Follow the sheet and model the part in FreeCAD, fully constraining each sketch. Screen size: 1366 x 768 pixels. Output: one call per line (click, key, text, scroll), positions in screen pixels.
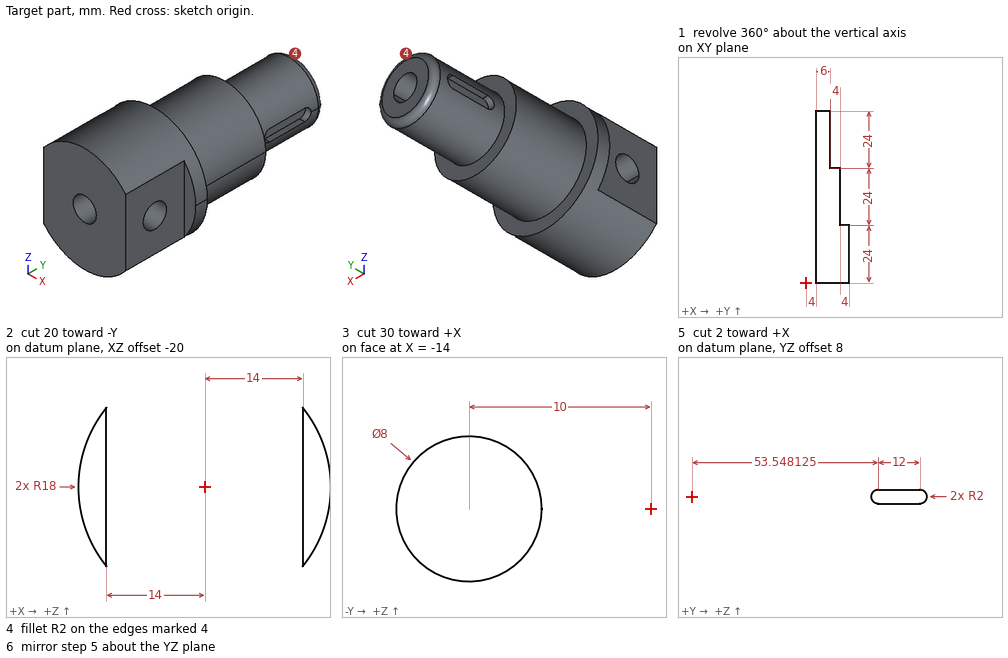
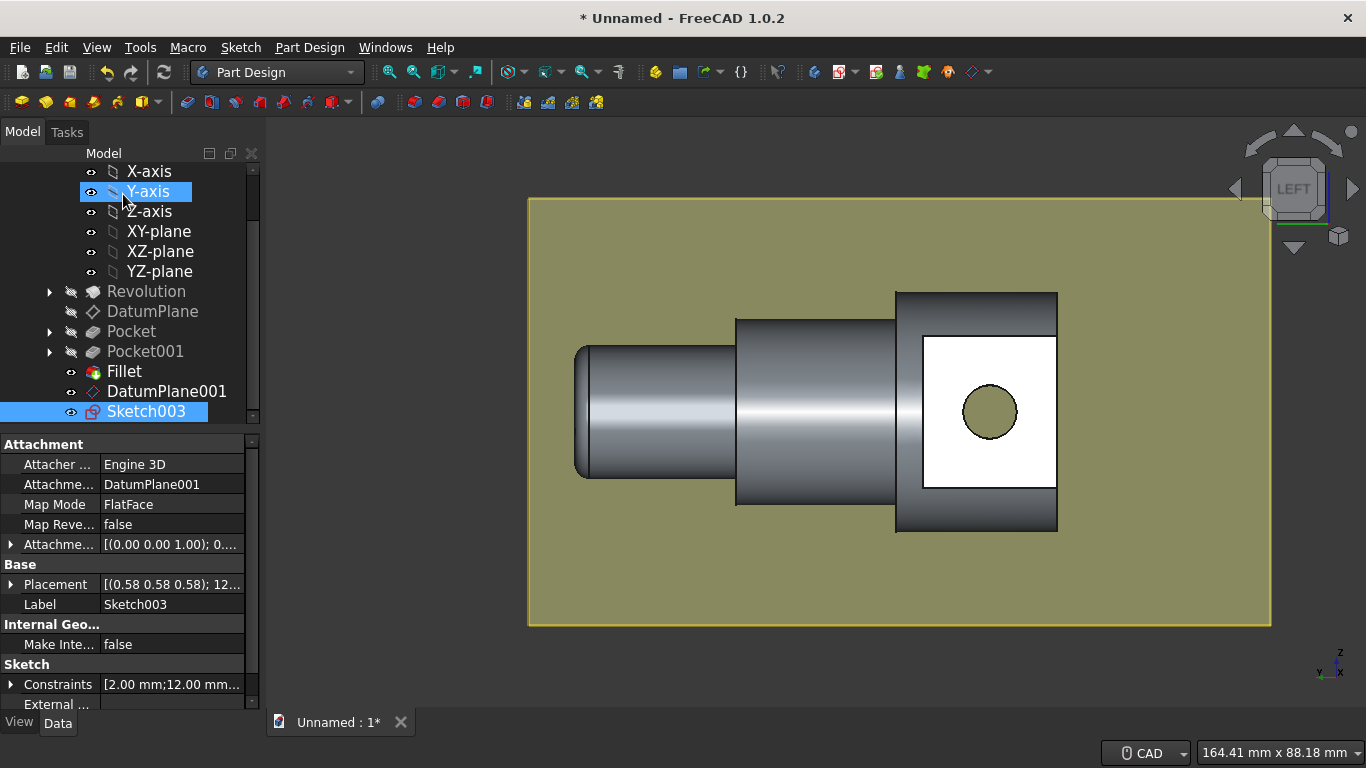
click(188, 102)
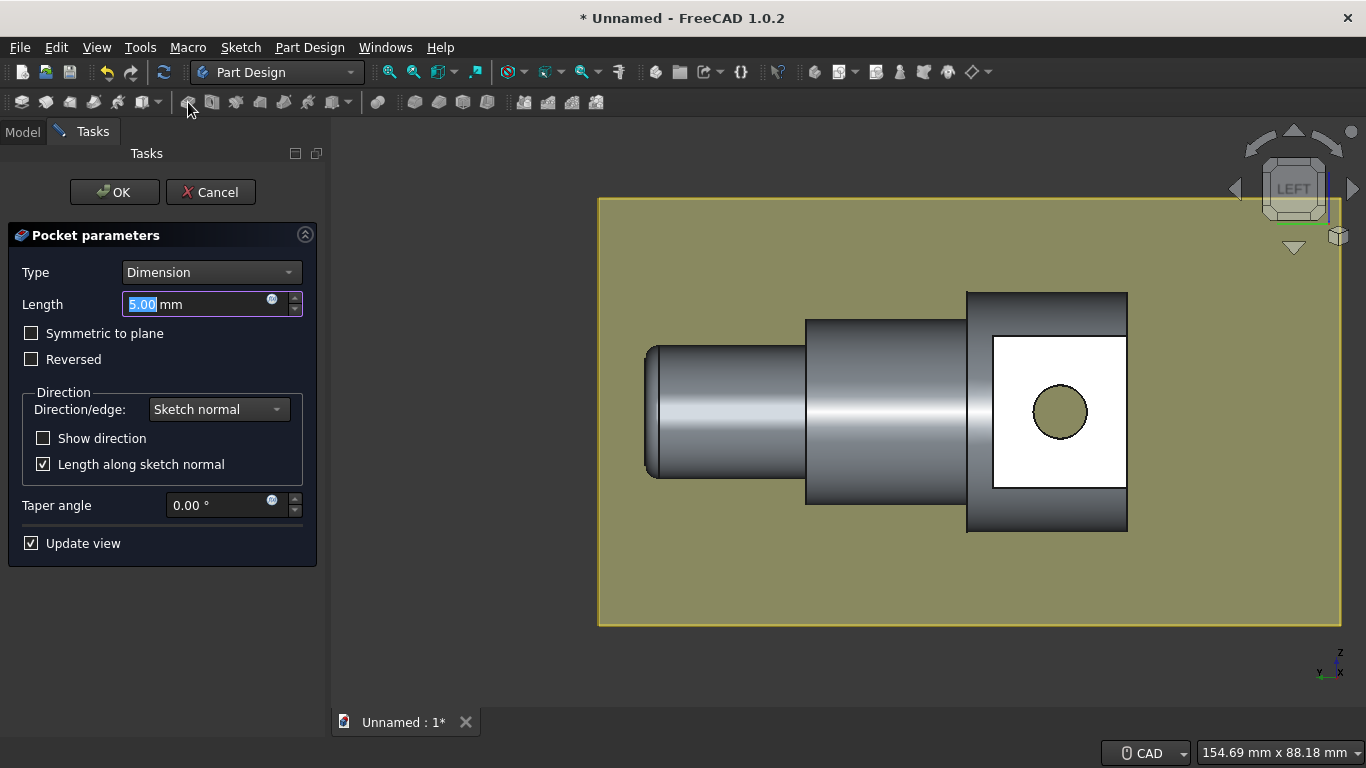
text(2)
key(Tab)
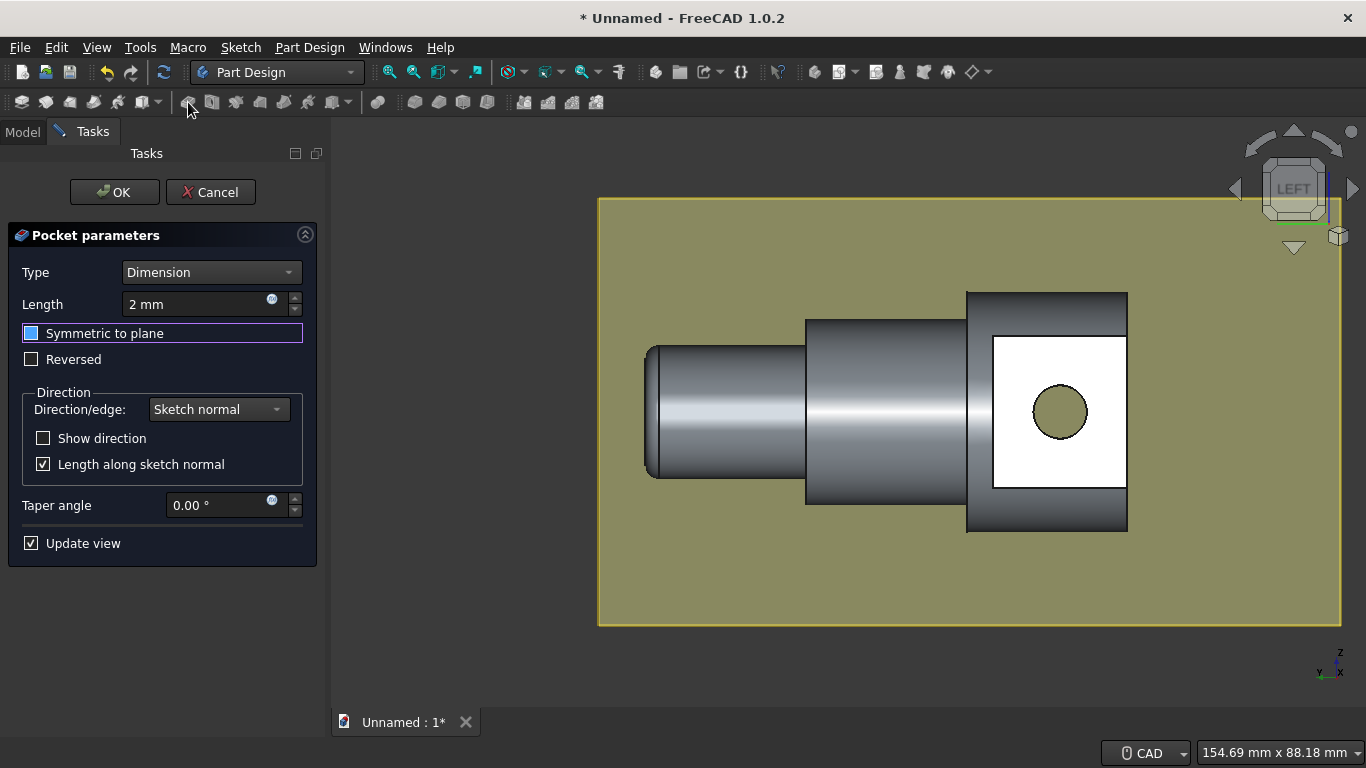
click(30, 359)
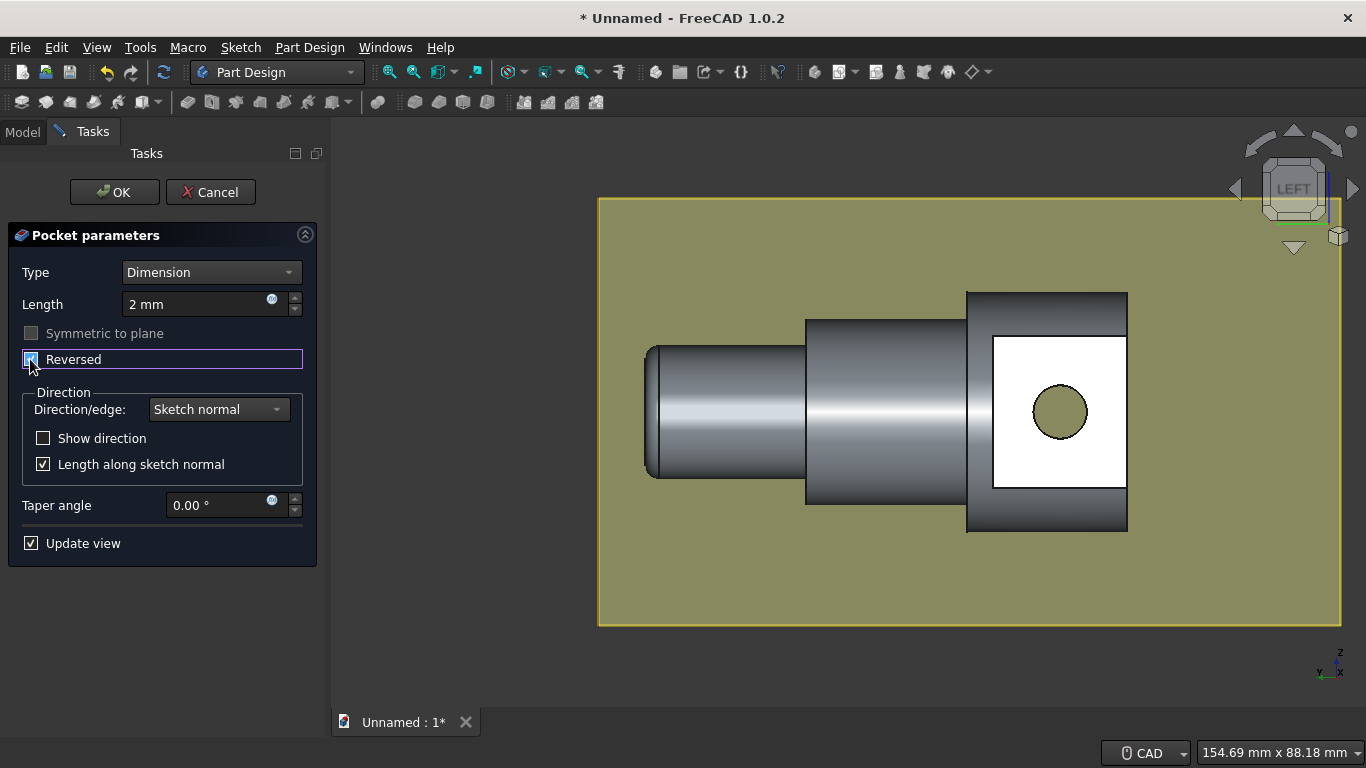
click(115, 192)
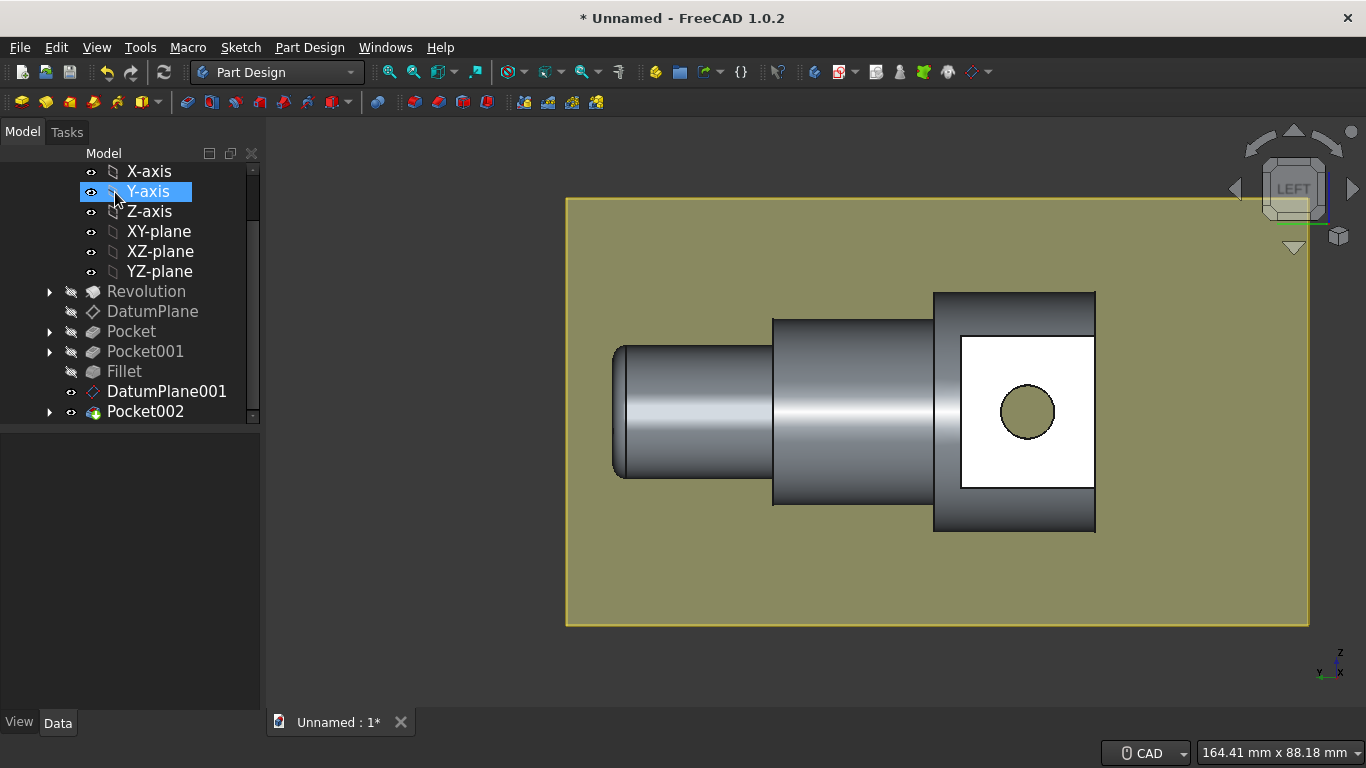
click(116, 392)
key(space)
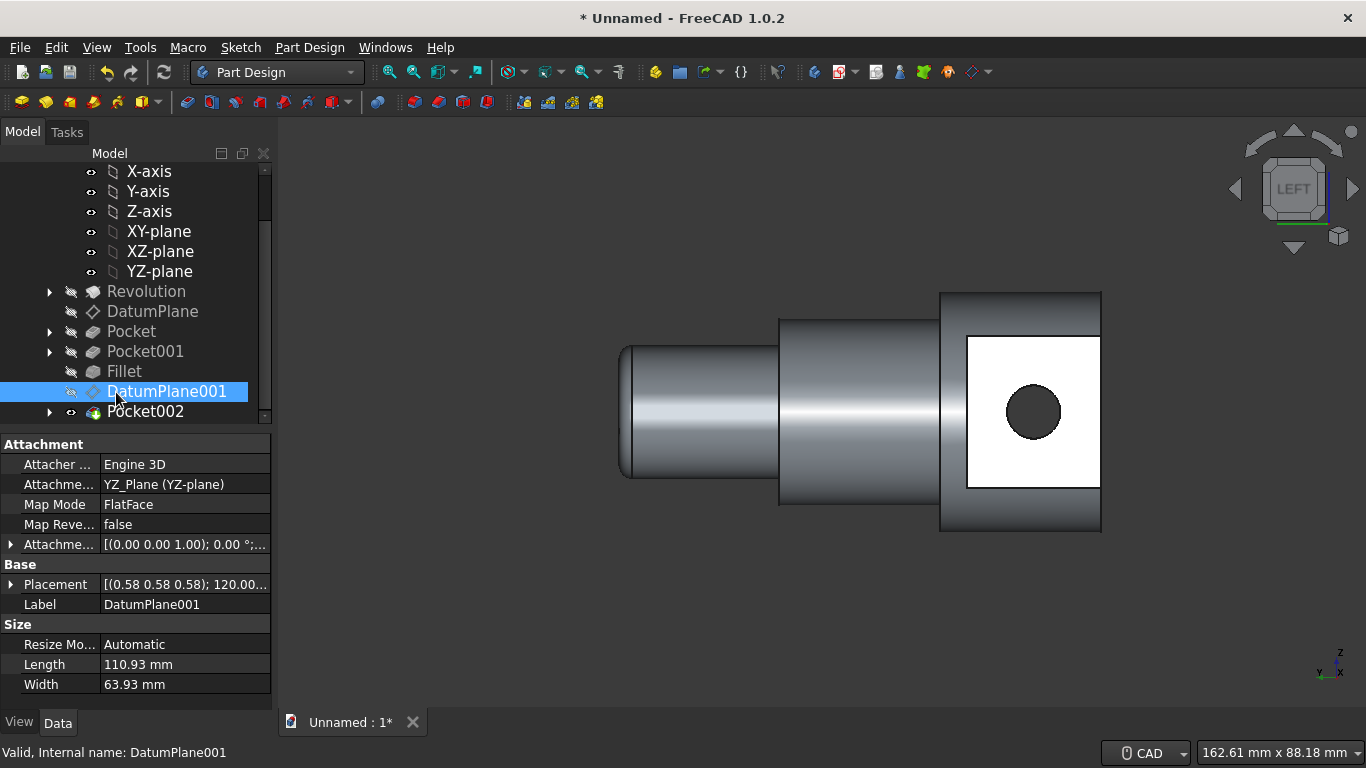
click(390, 72)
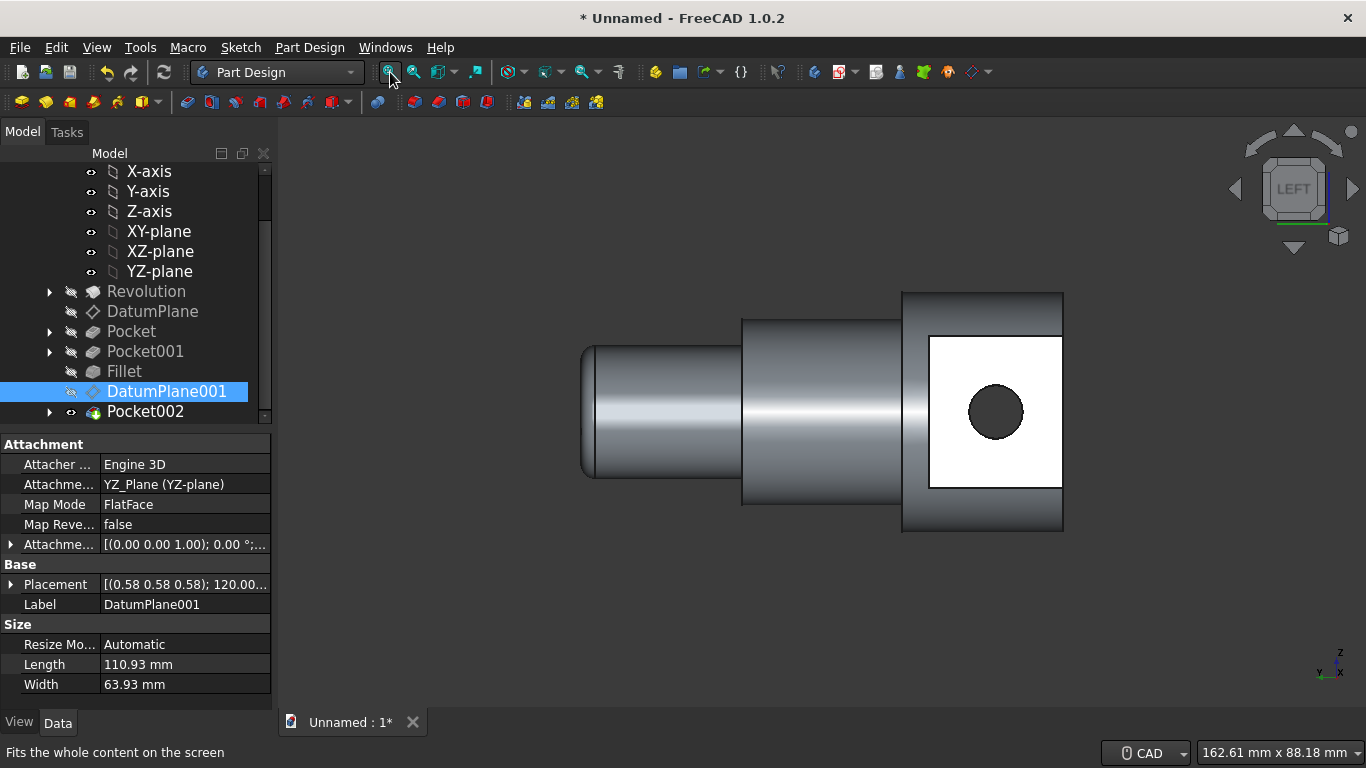
click(116, 412)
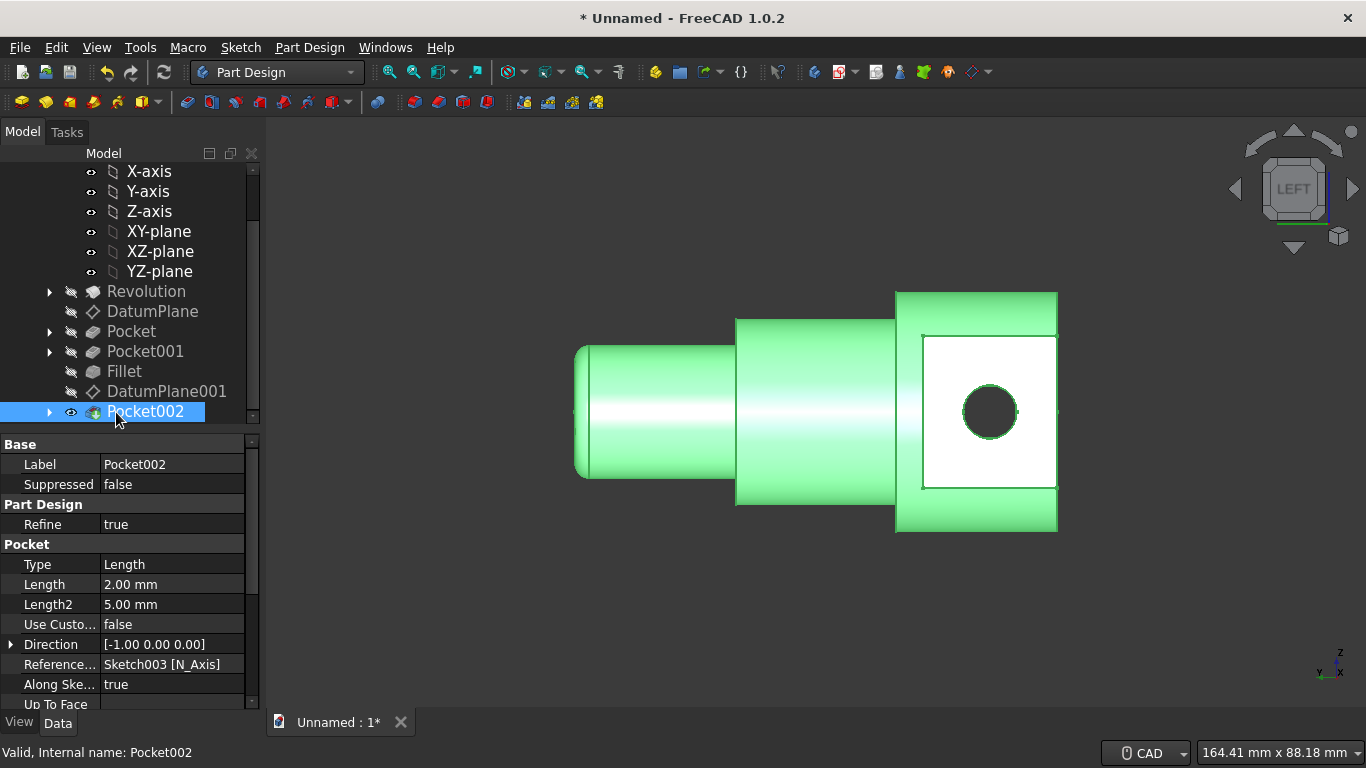
click(524, 102)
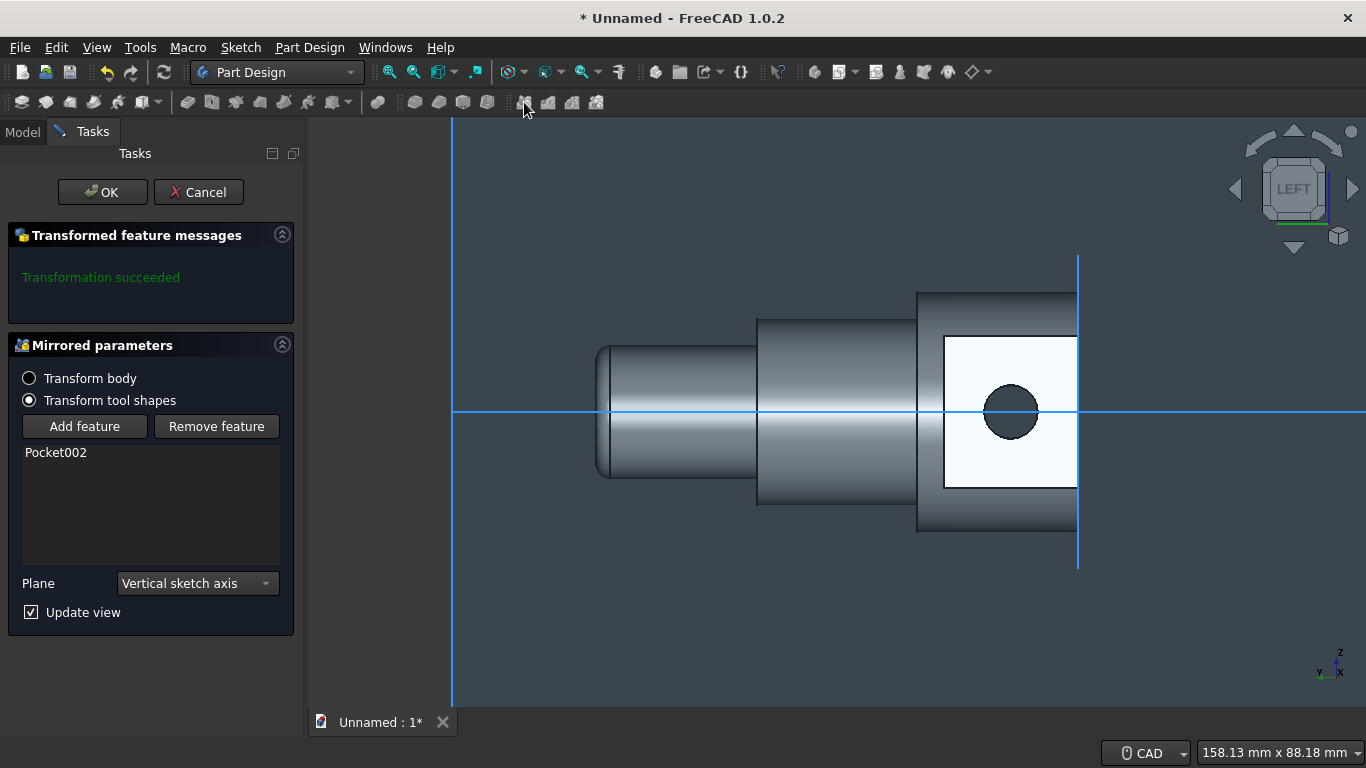
click(198, 584)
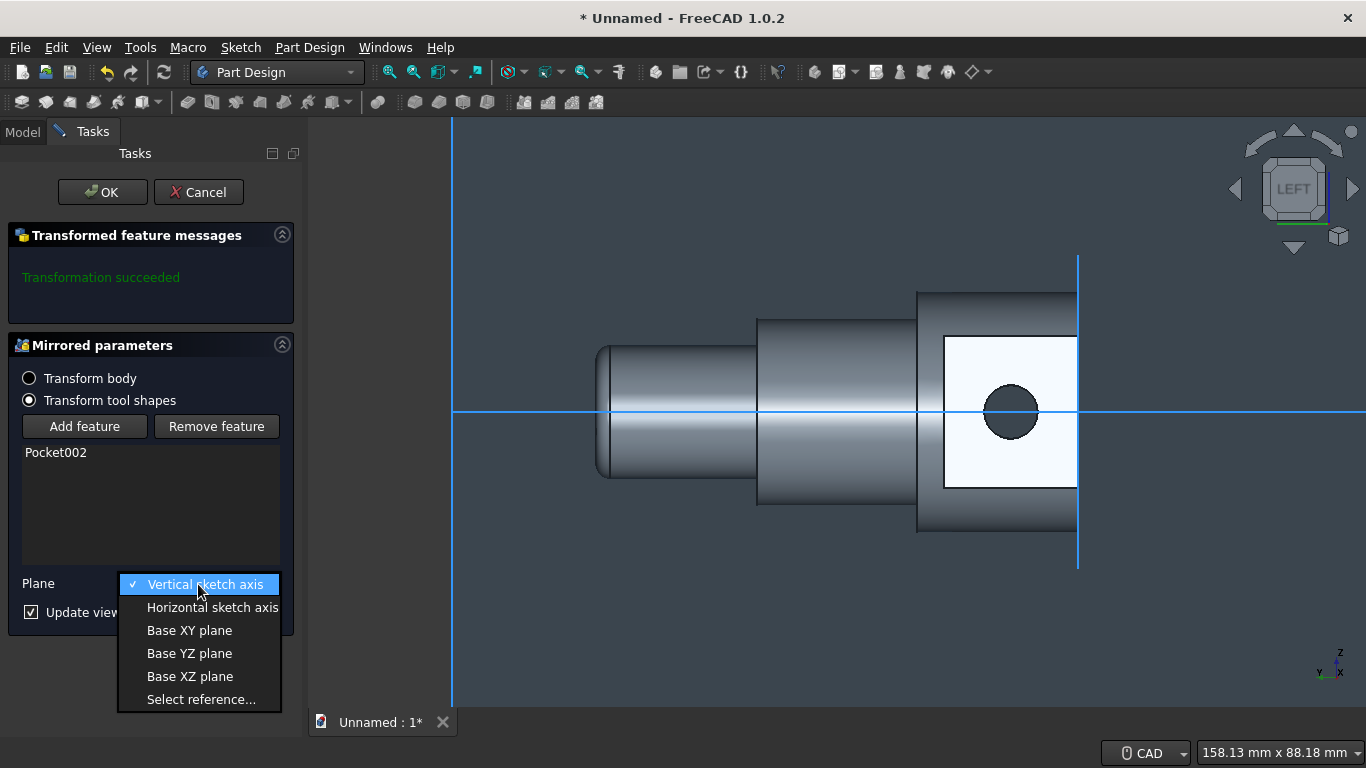
click(198, 654)